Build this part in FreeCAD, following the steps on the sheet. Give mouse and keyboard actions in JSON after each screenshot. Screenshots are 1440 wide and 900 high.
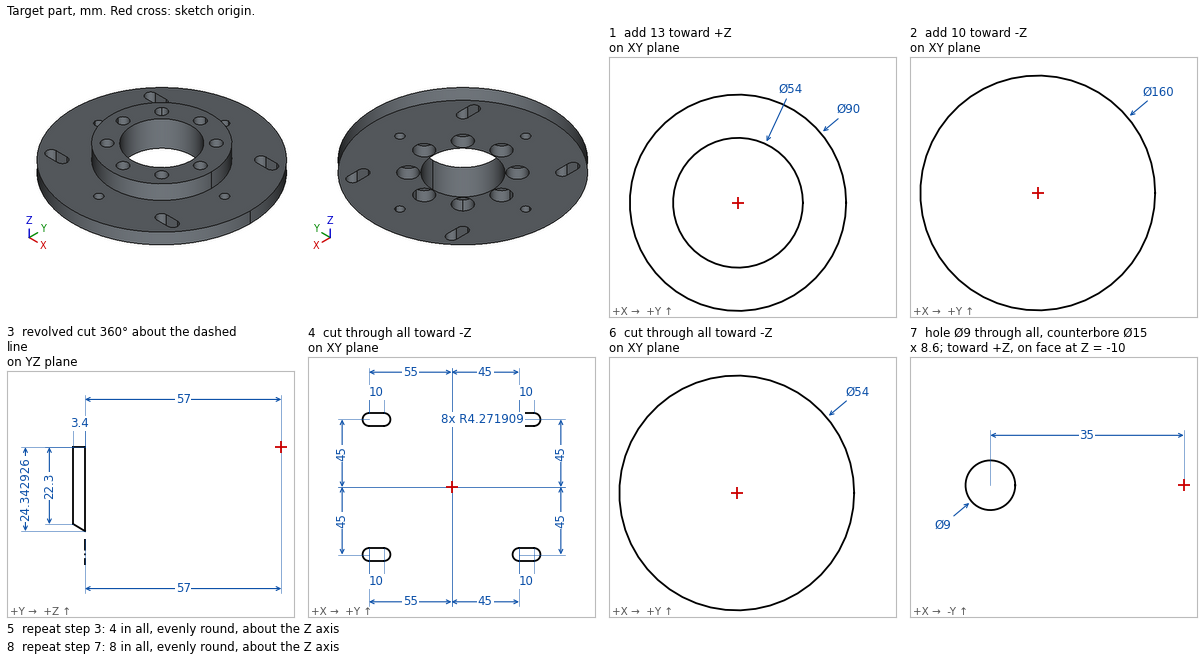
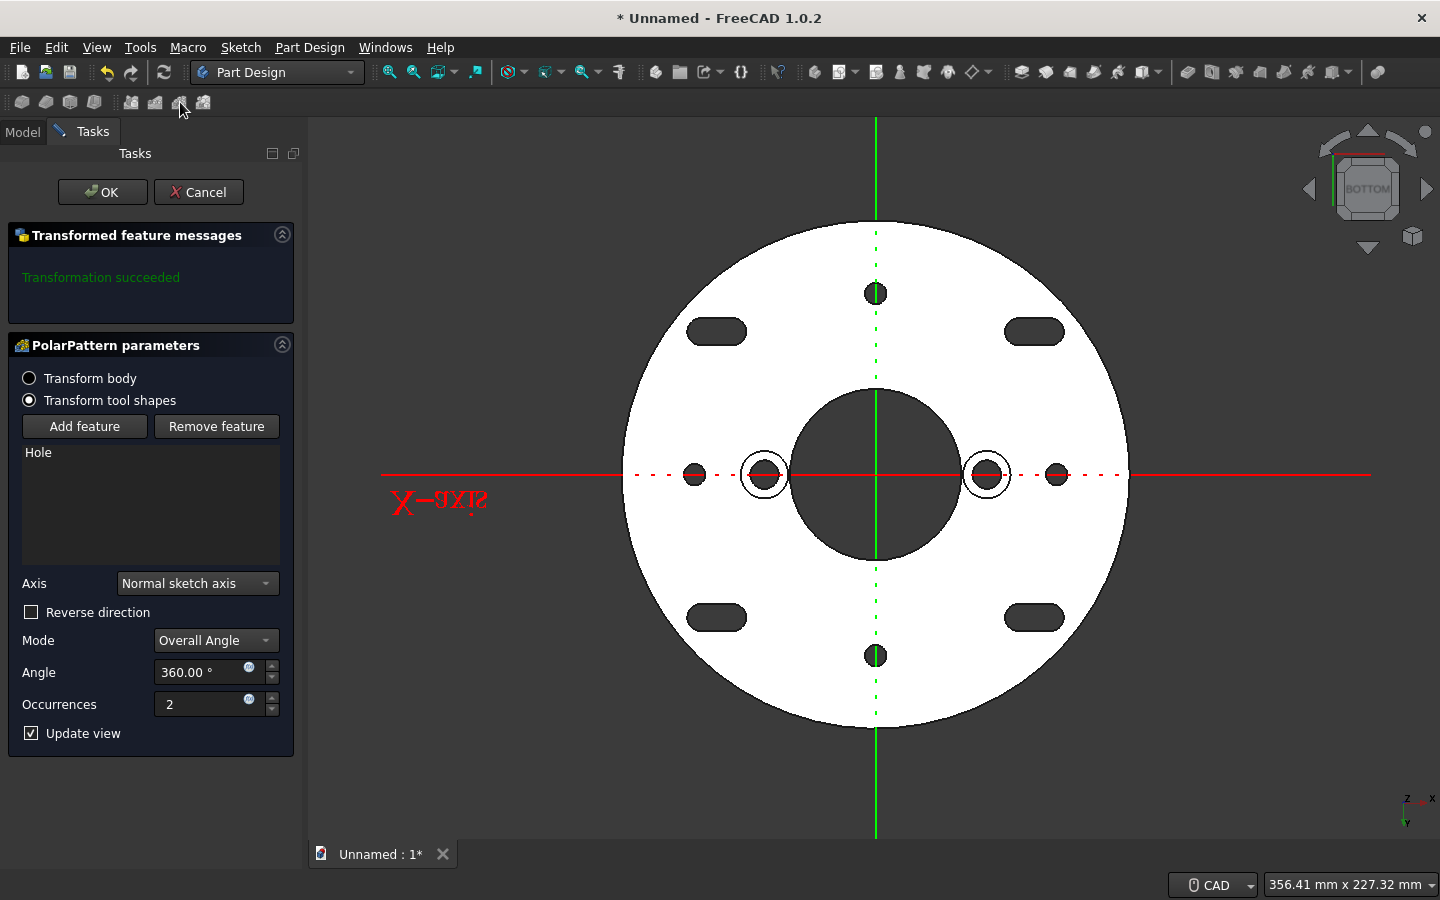
{"action": "left_click", "coordinate": [198, 584]}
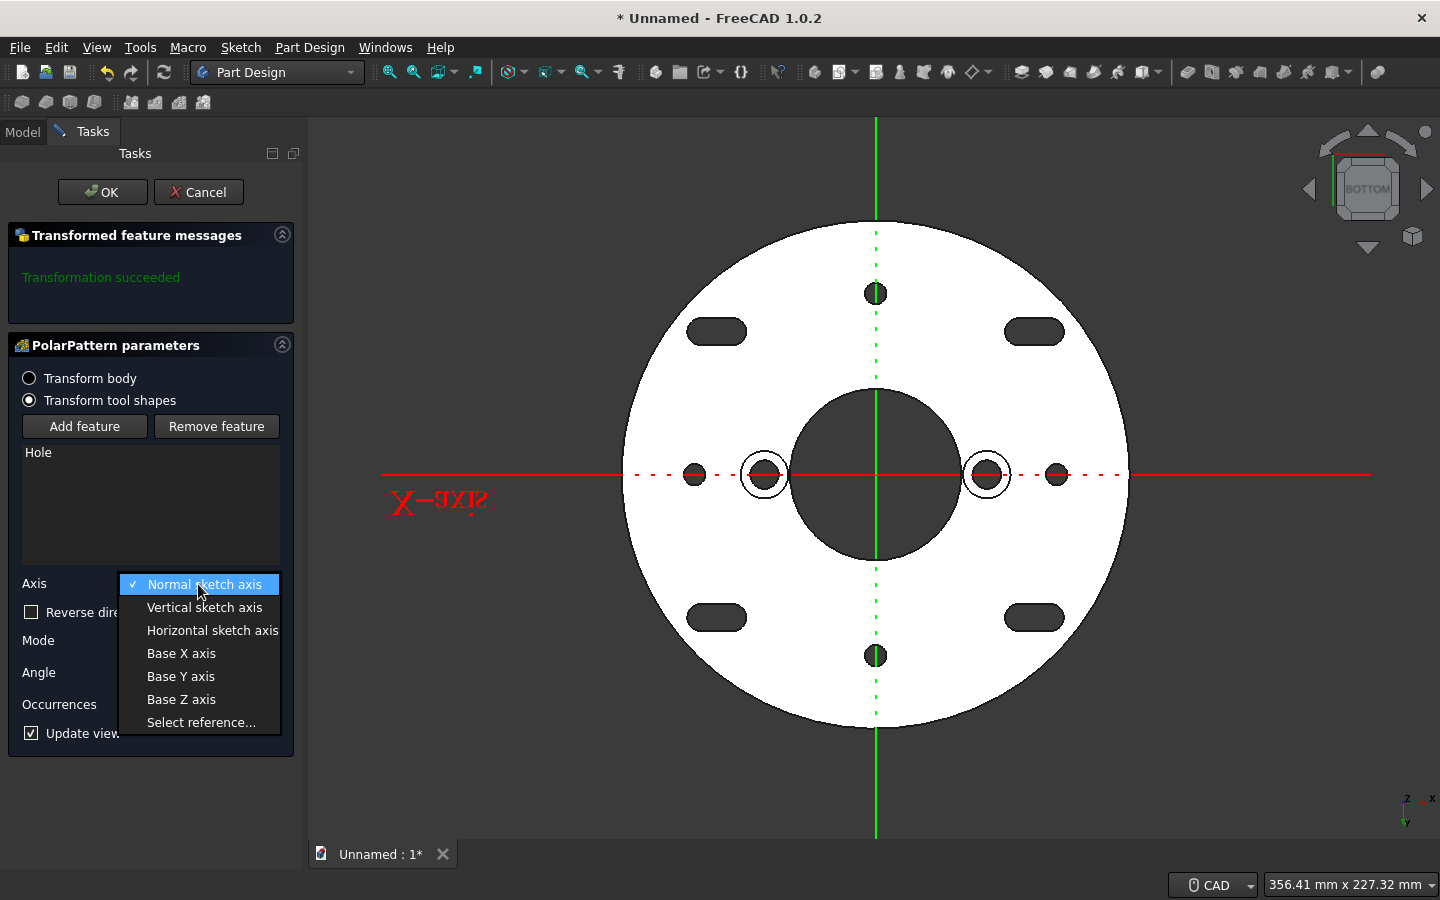
{"action": "left_click", "coordinate": [198, 700]}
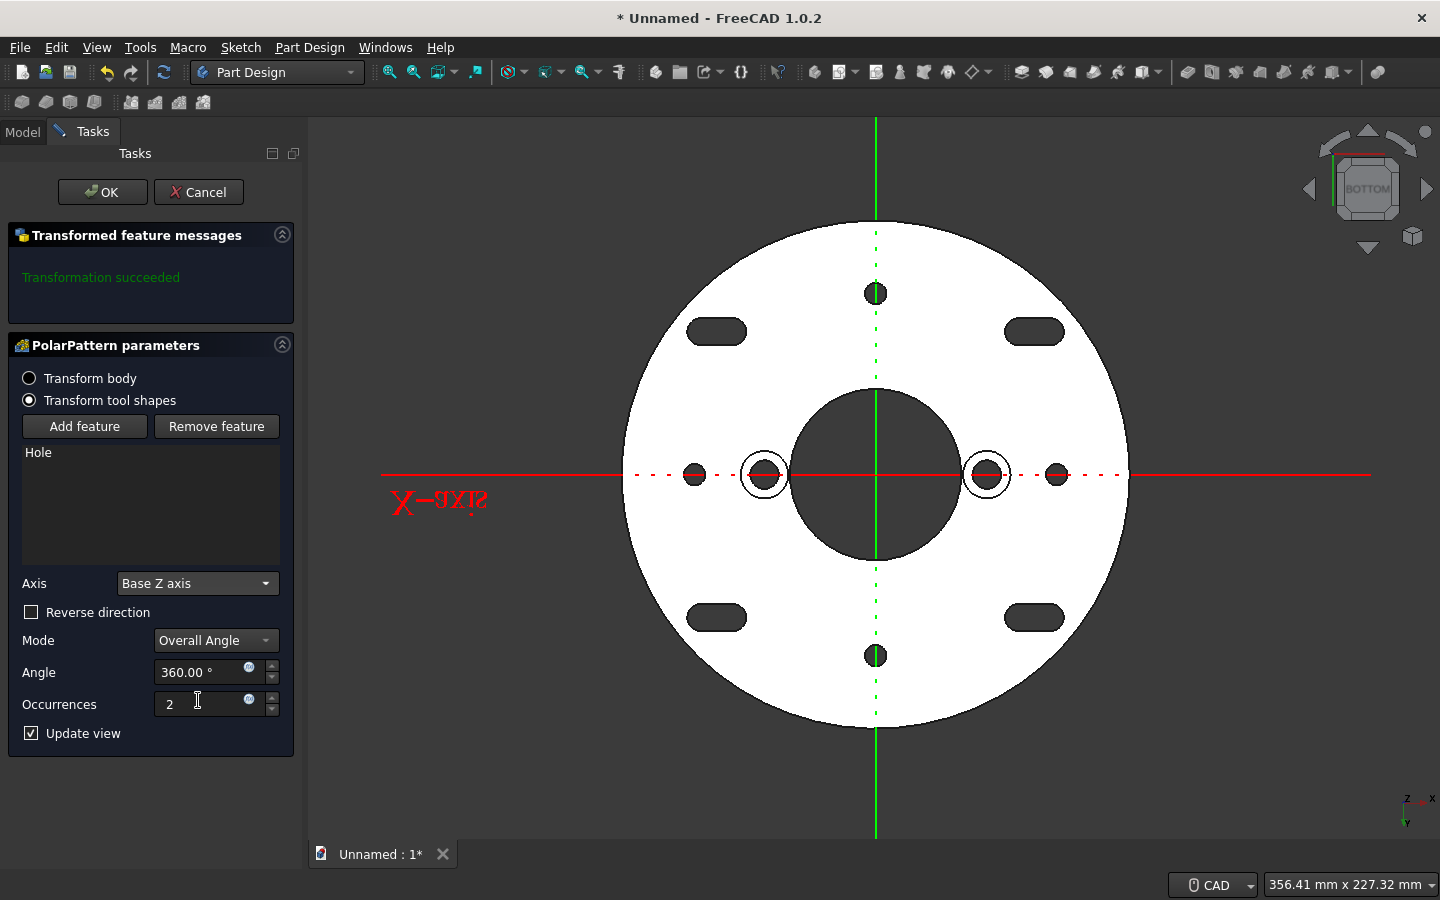
{"action": "triple_click", "coordinate": [209, 704]}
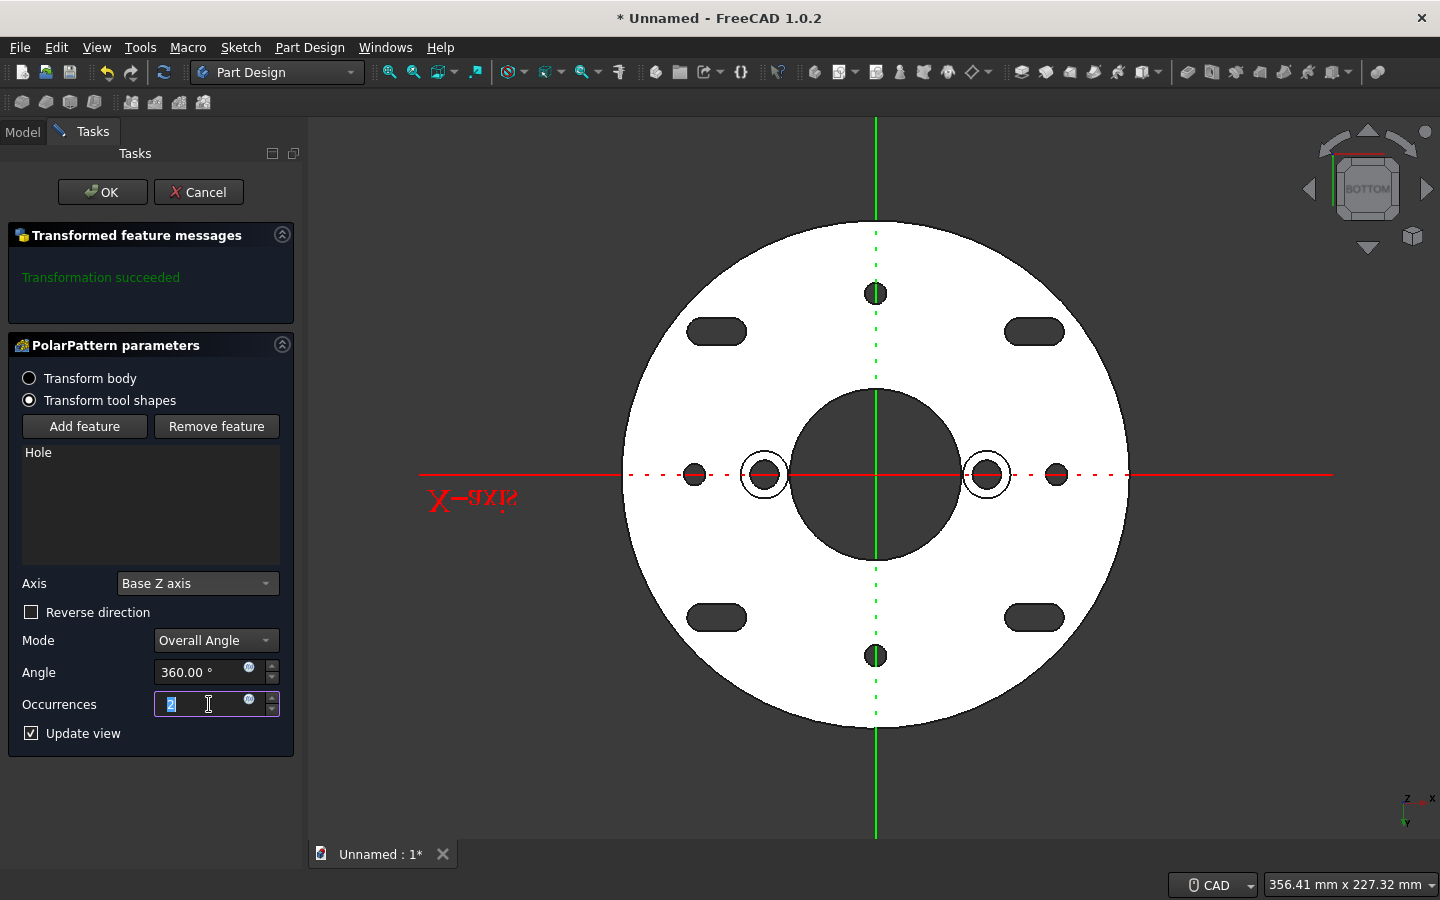
{"action": "type", "text": "8"}
{"action": "key", "text": "Tab"}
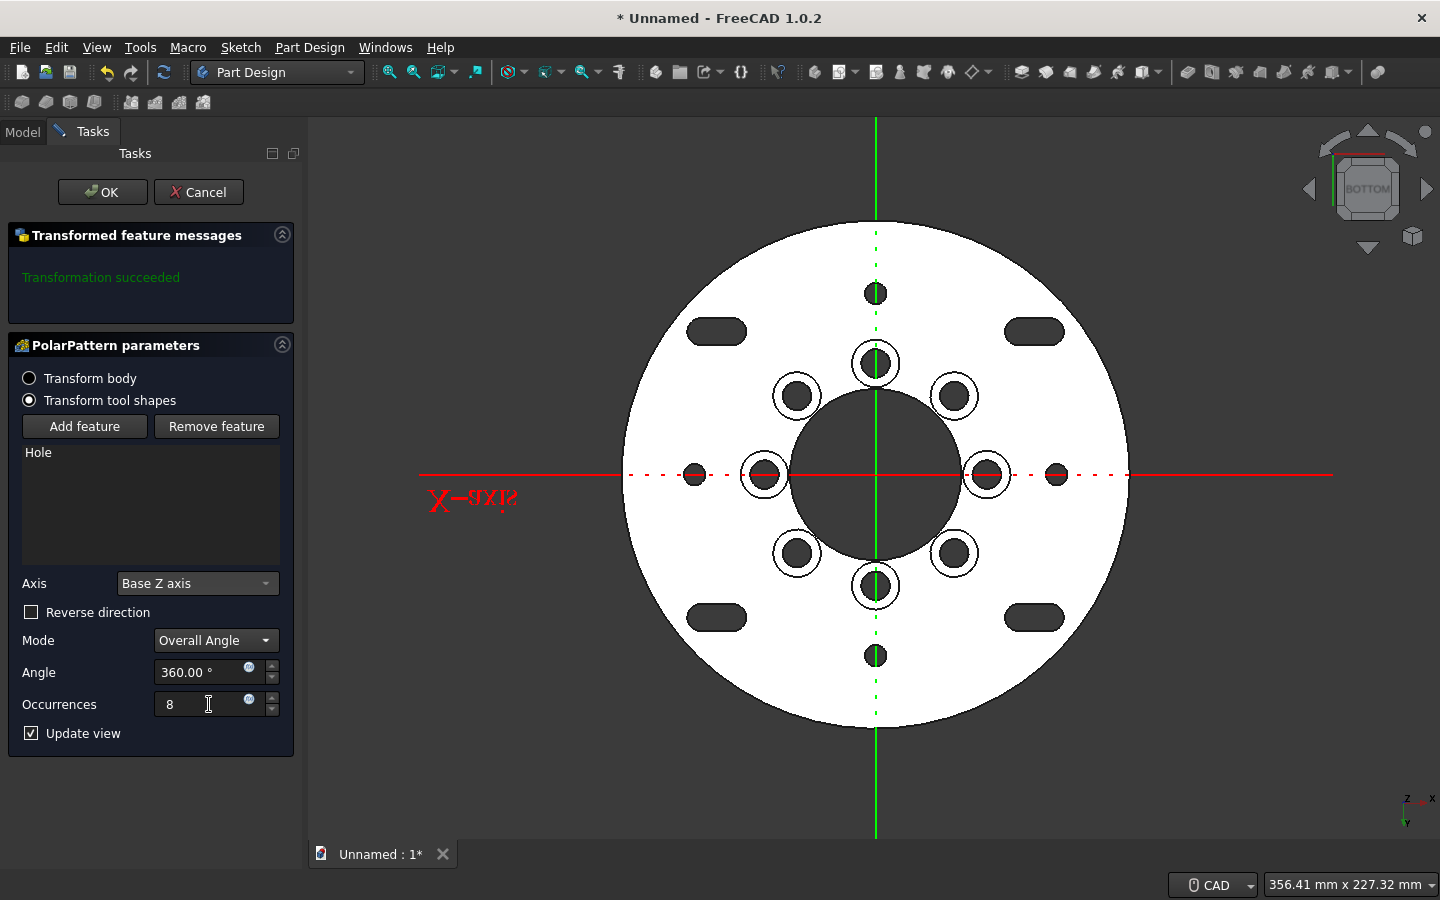
{"action": "left_click", "coordinate": [103, 192]}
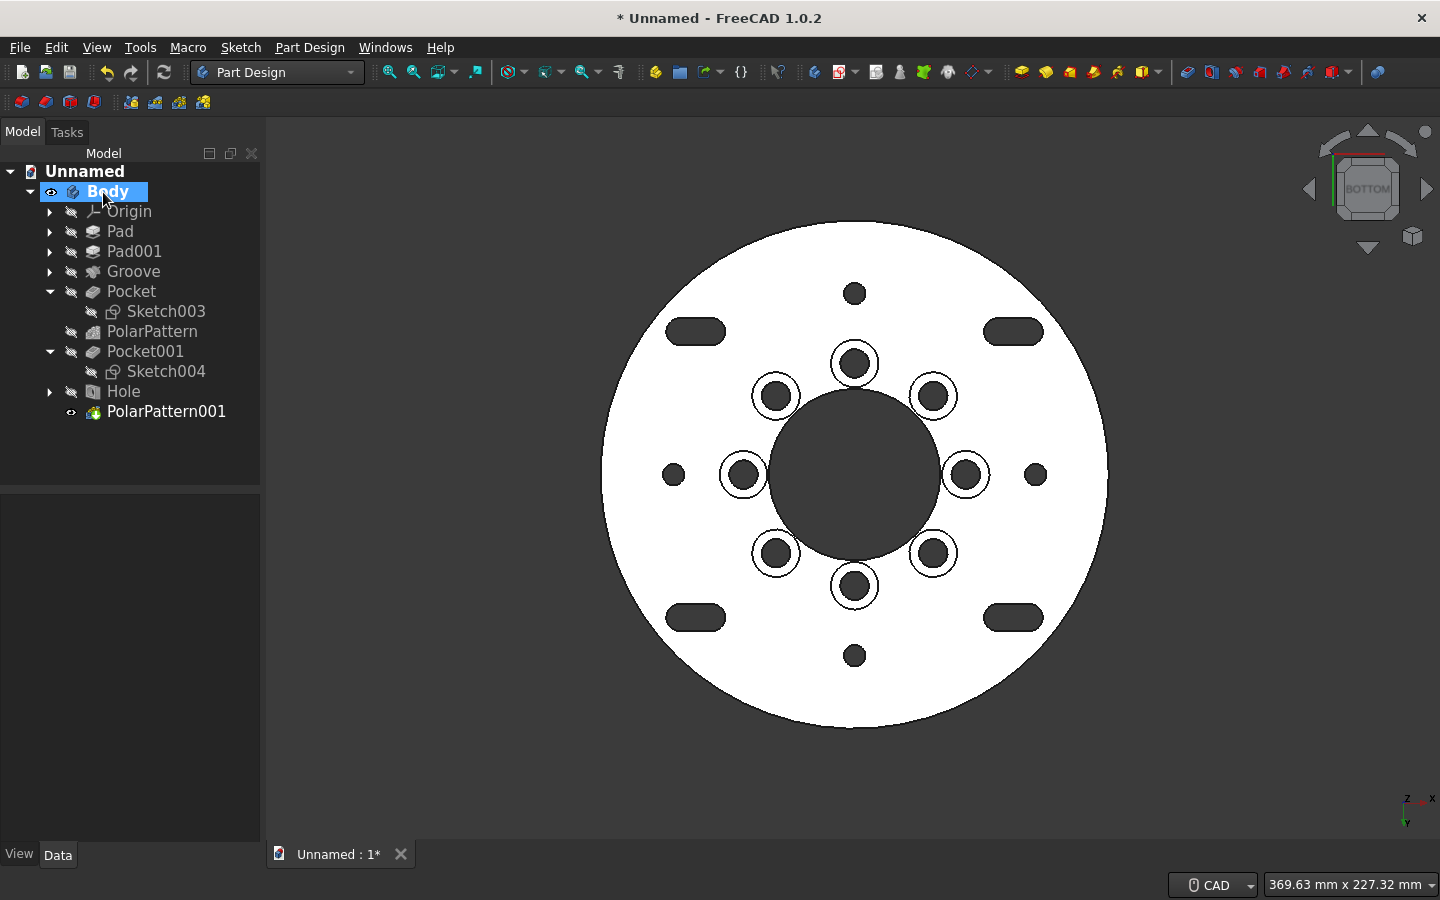
{"action": "key", "text": "0"}